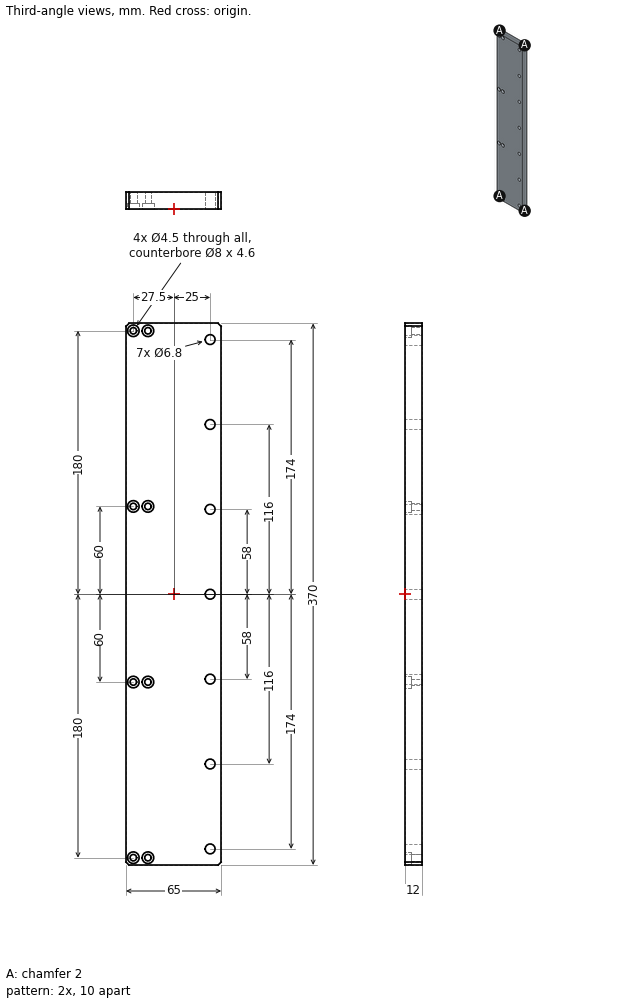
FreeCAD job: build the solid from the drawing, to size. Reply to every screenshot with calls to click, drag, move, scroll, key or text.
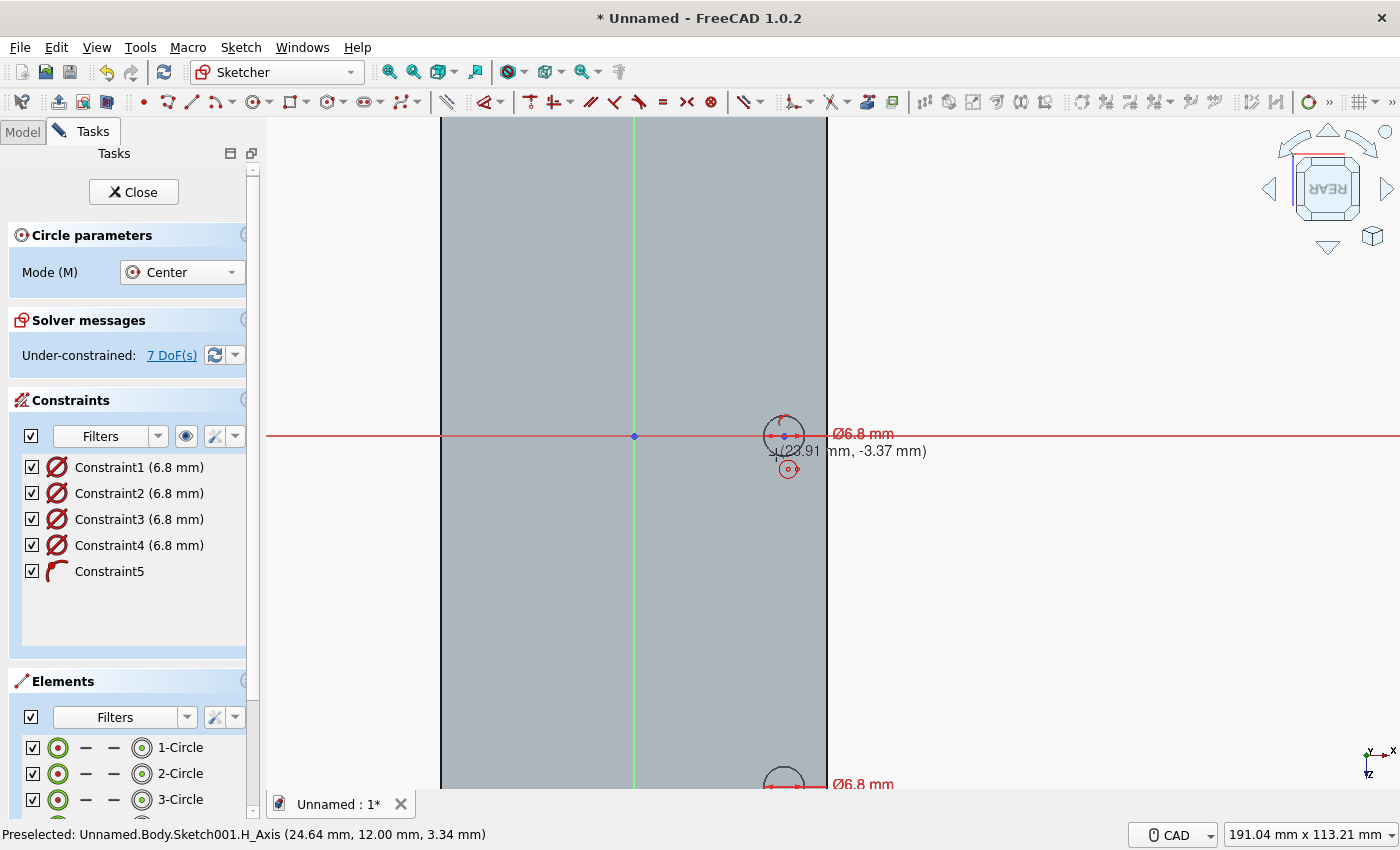
scroll(776, 457, down, 8)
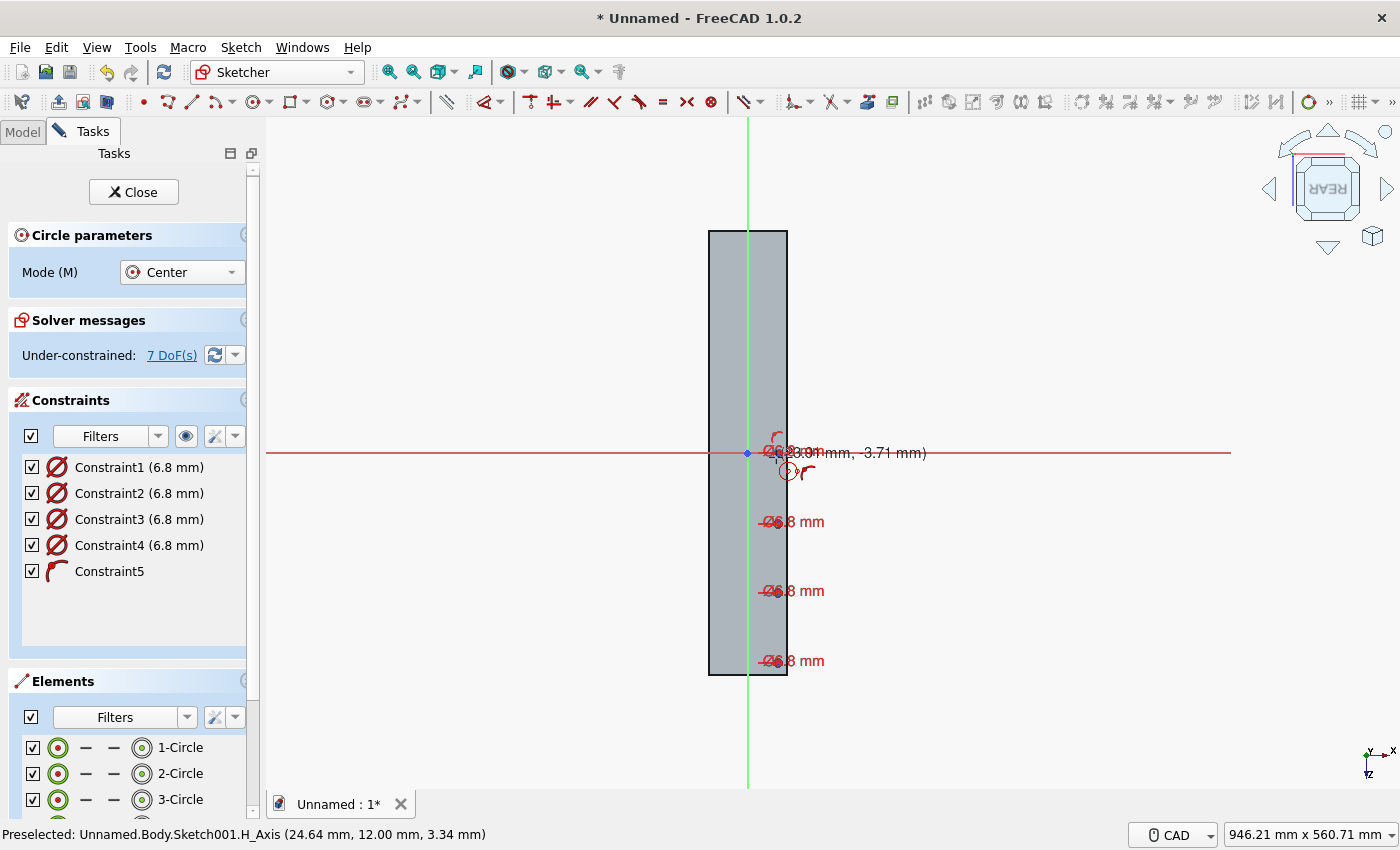
scroll(778, 384, up, 9)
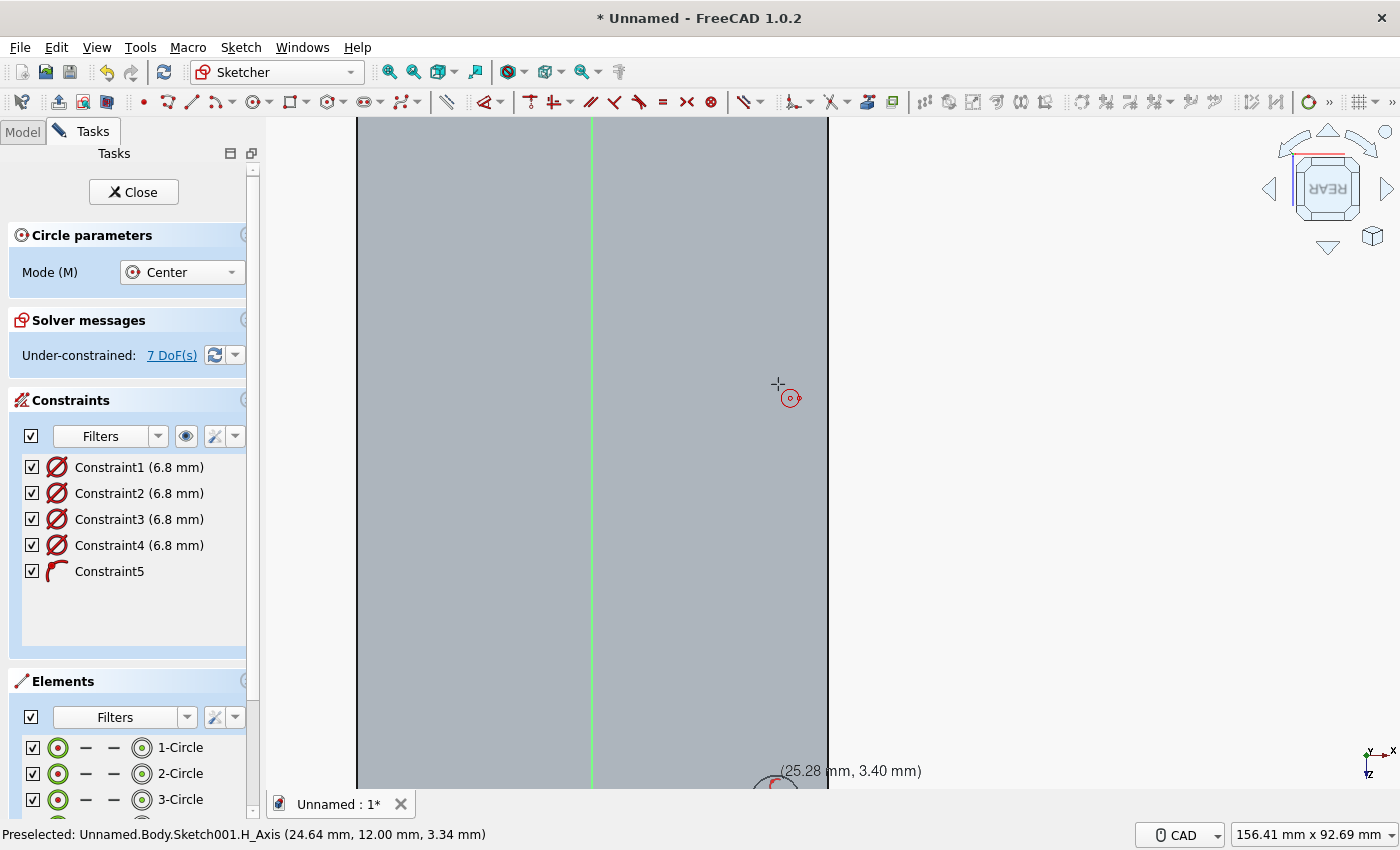
scroll(778, 384, down, 9)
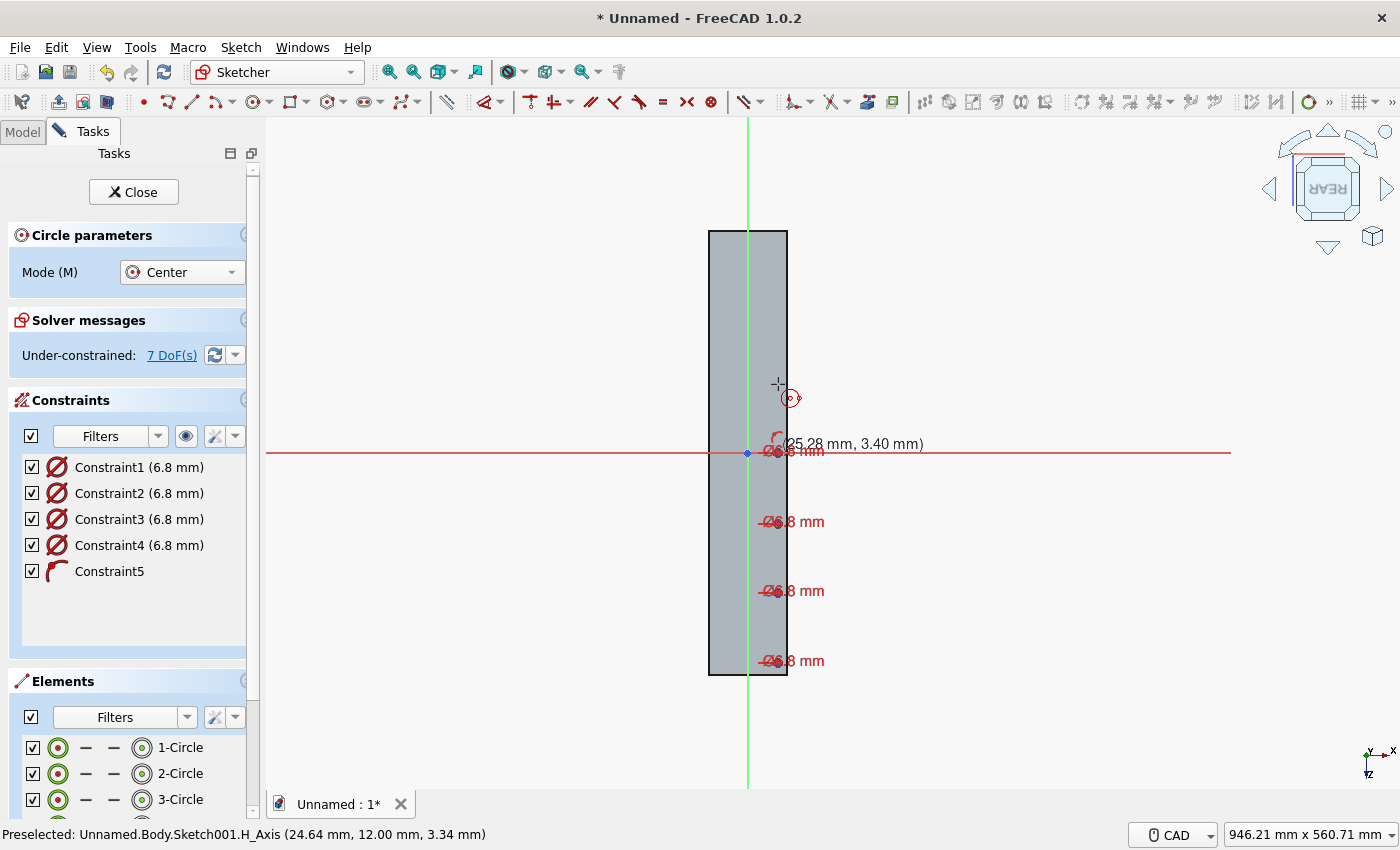
click(778, 384)
move(781, 381)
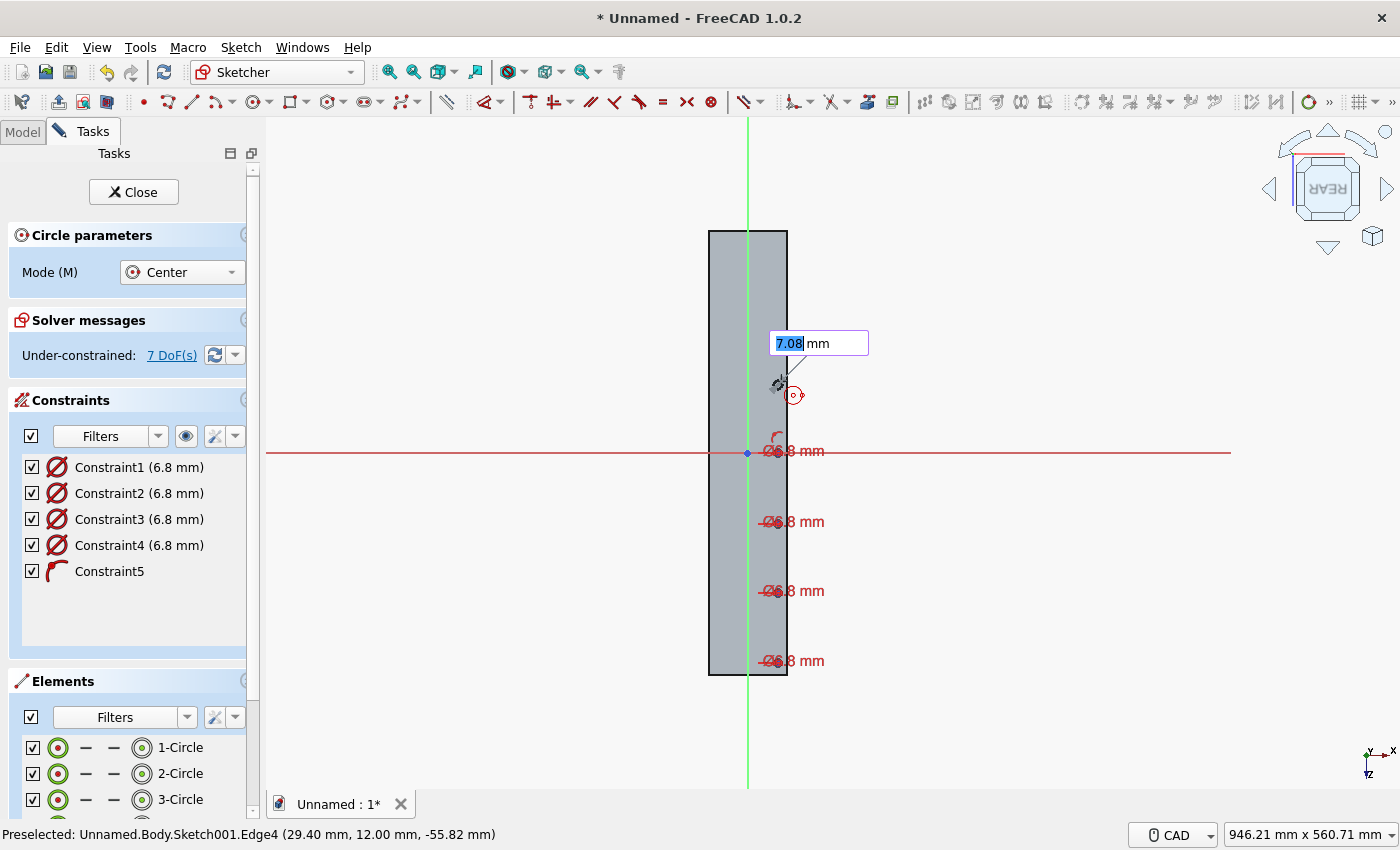
text(6.8)
key(Return)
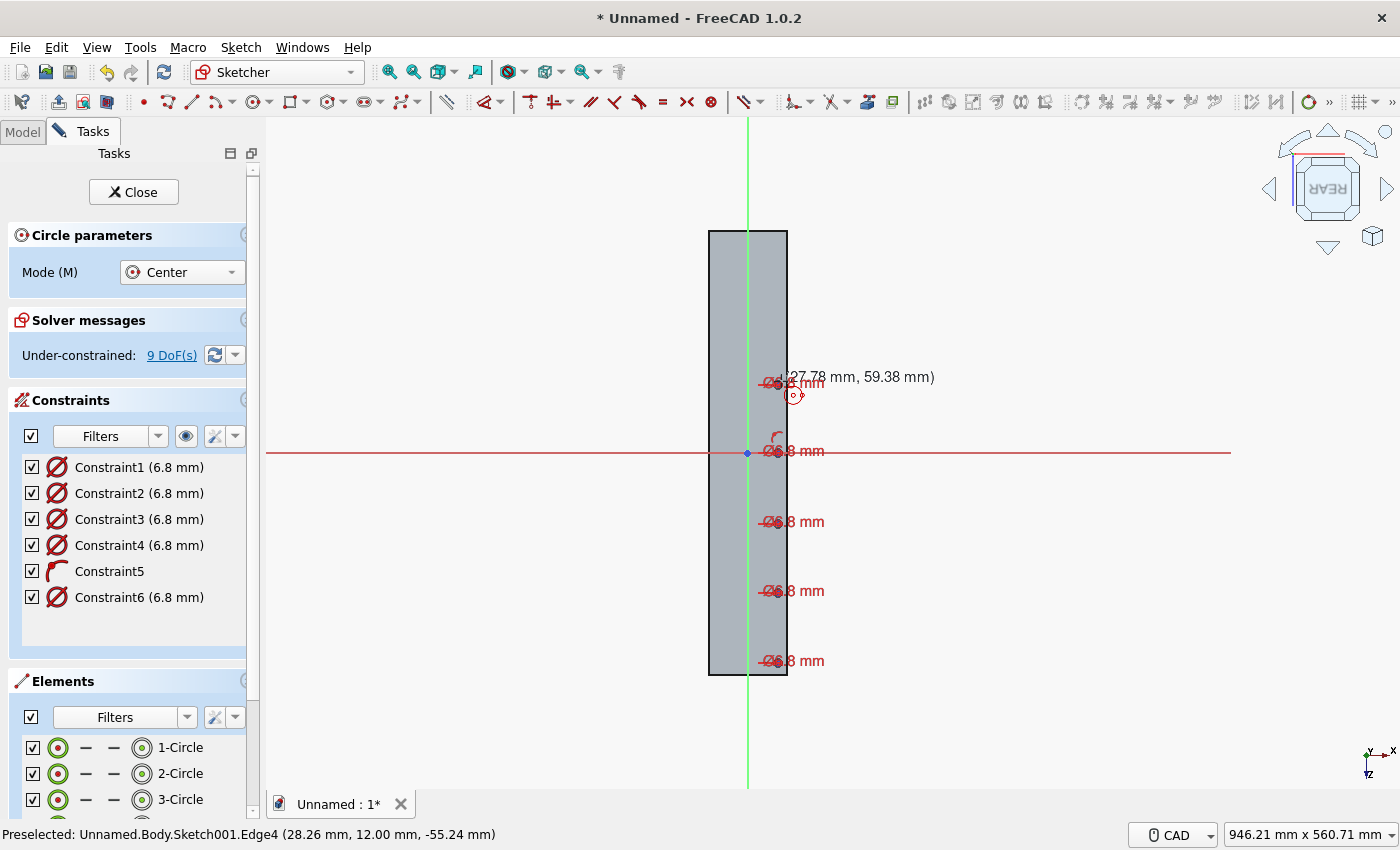
scroll(778, 314, up, 9)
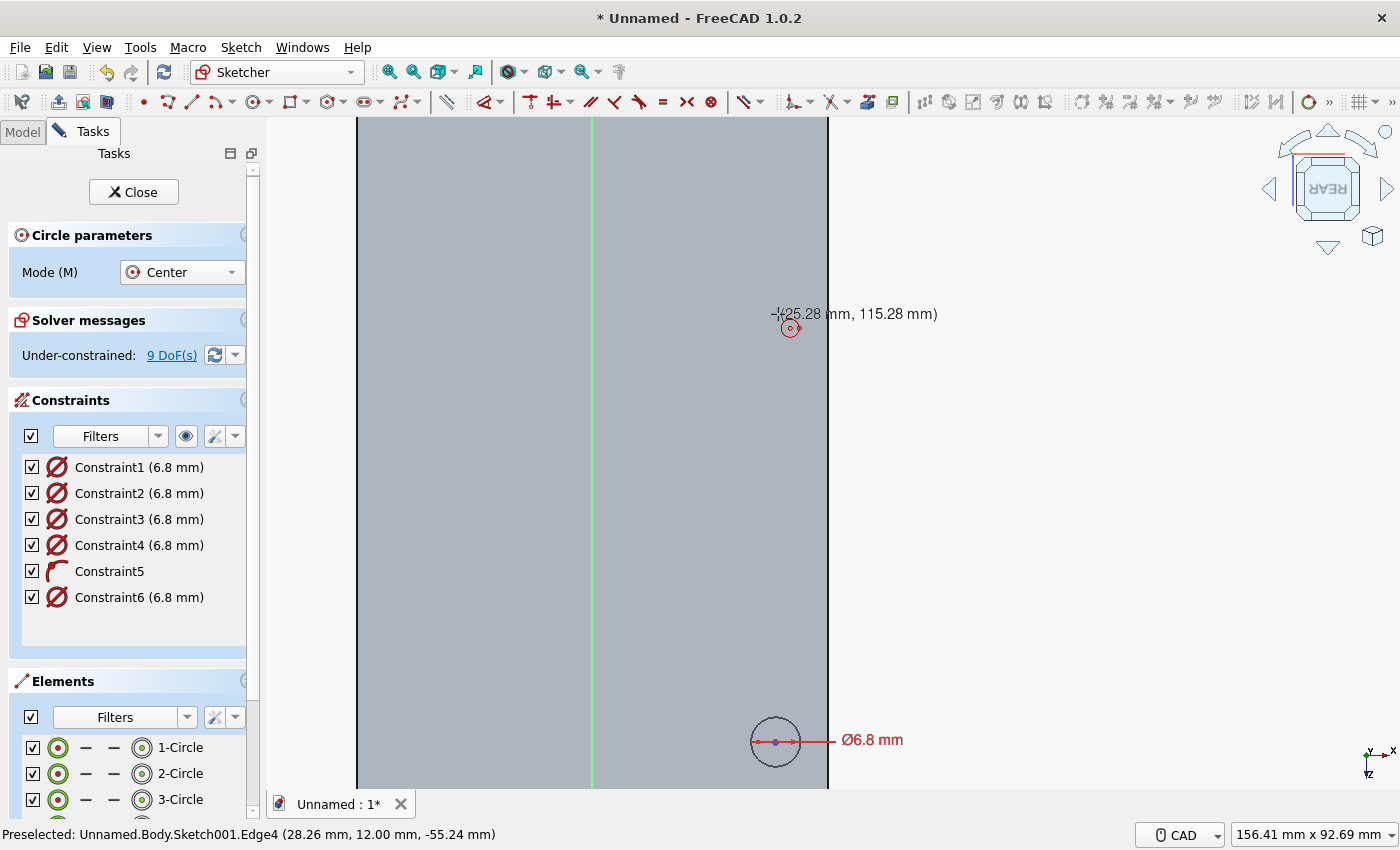
scroll(778, 314, down, 9)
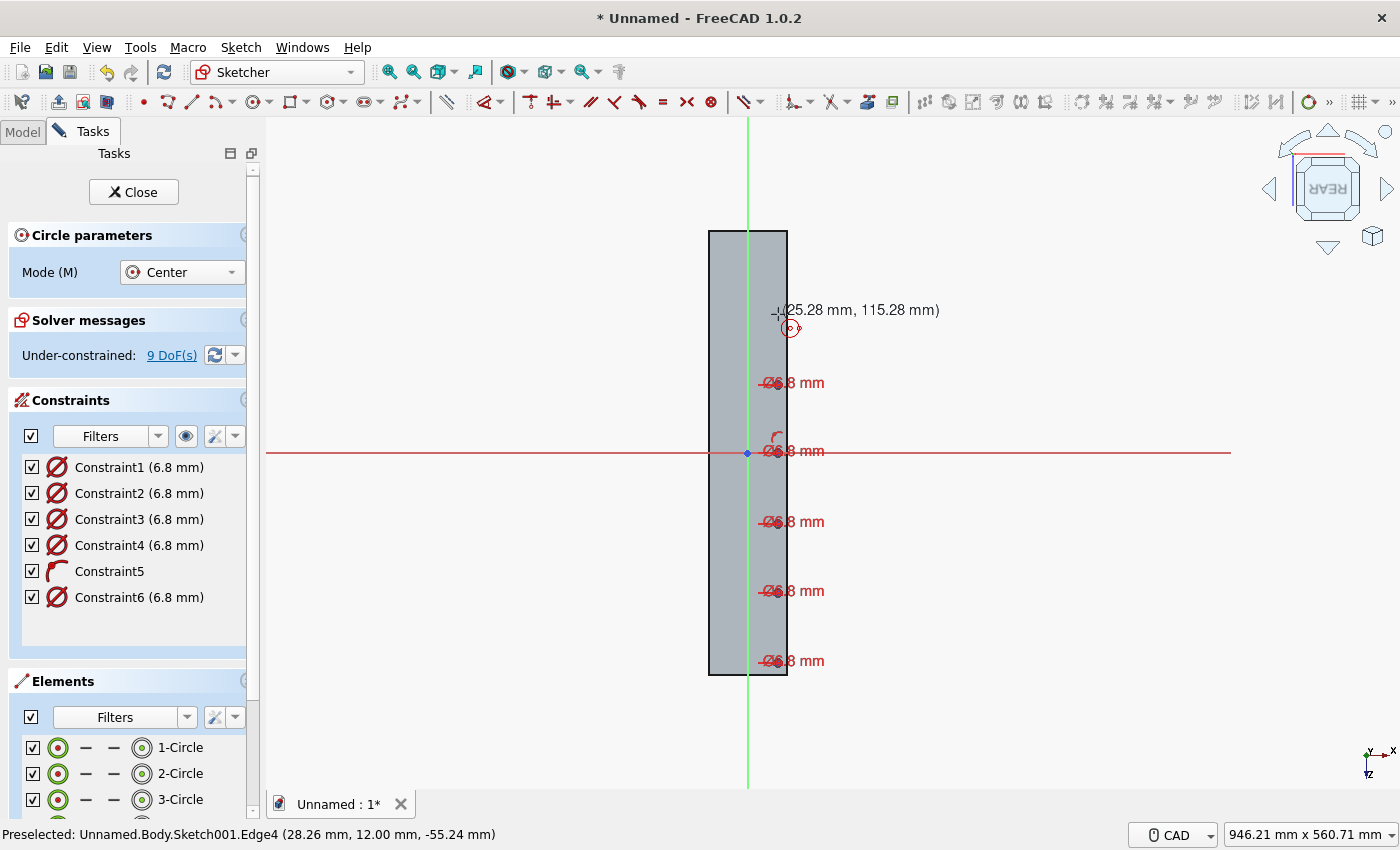
click(778, 314)
move(781, 311)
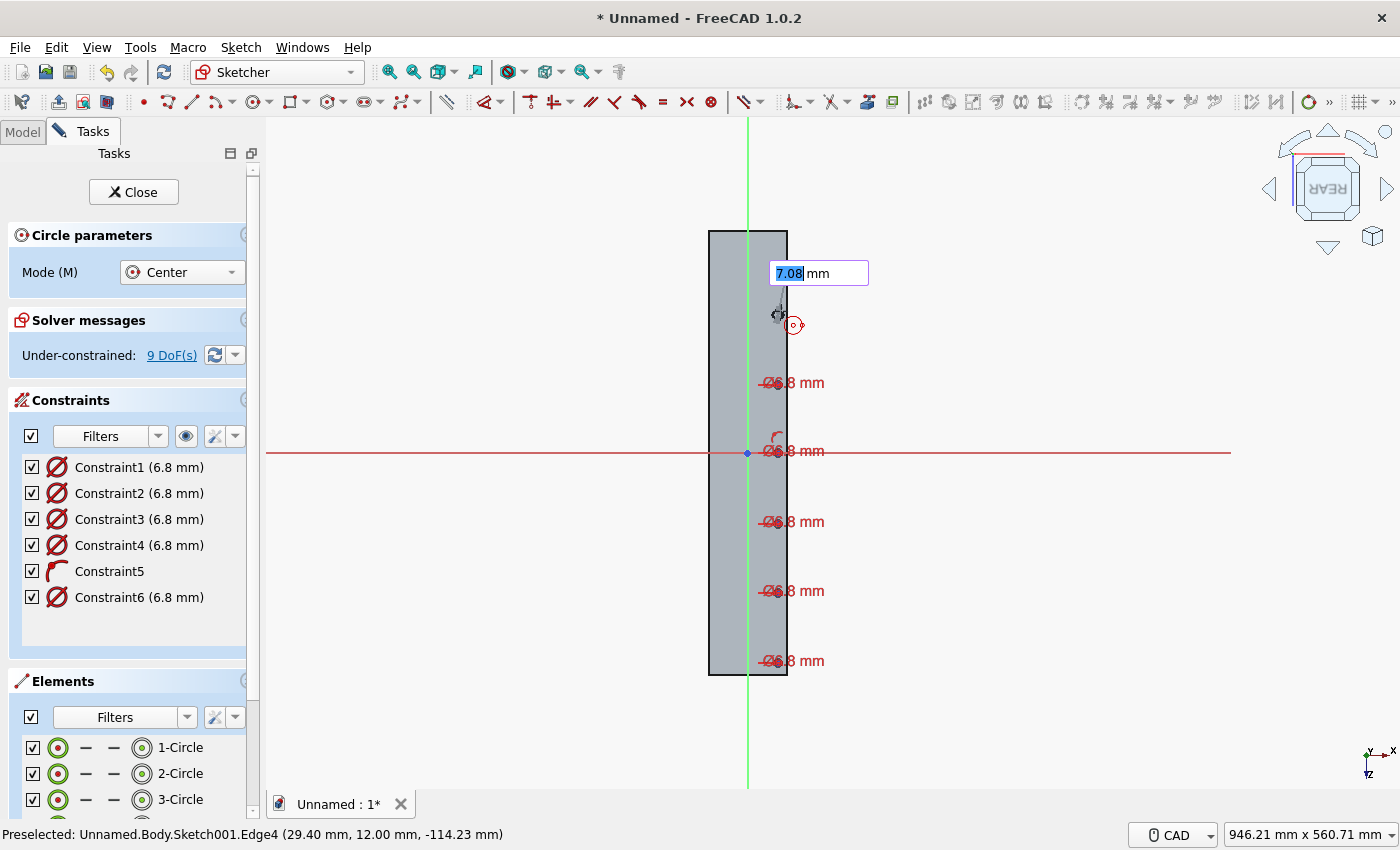
text(6.8)
key(Return)